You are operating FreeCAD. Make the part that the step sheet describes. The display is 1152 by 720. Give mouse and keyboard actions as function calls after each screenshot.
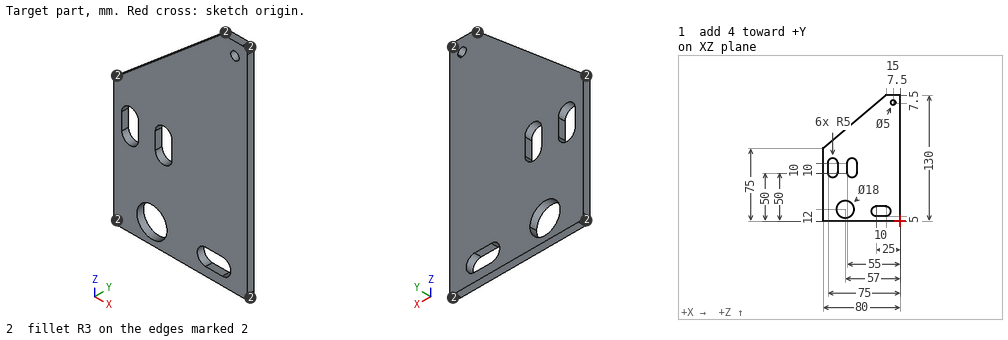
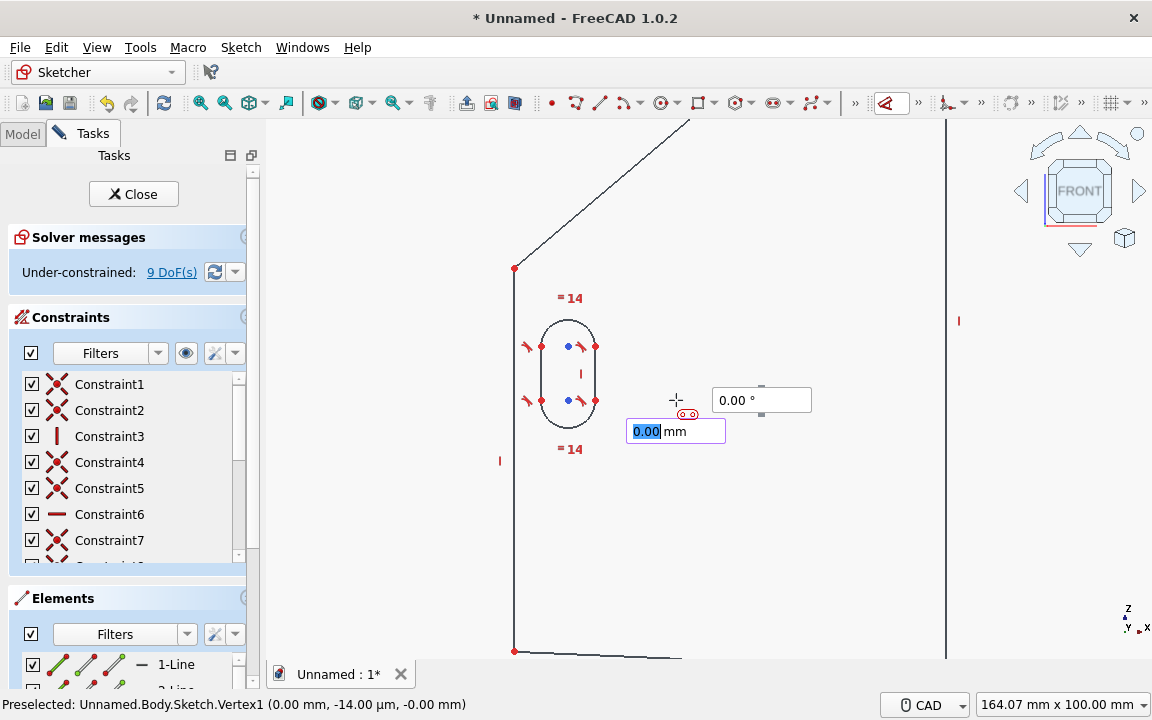
click(676, 346)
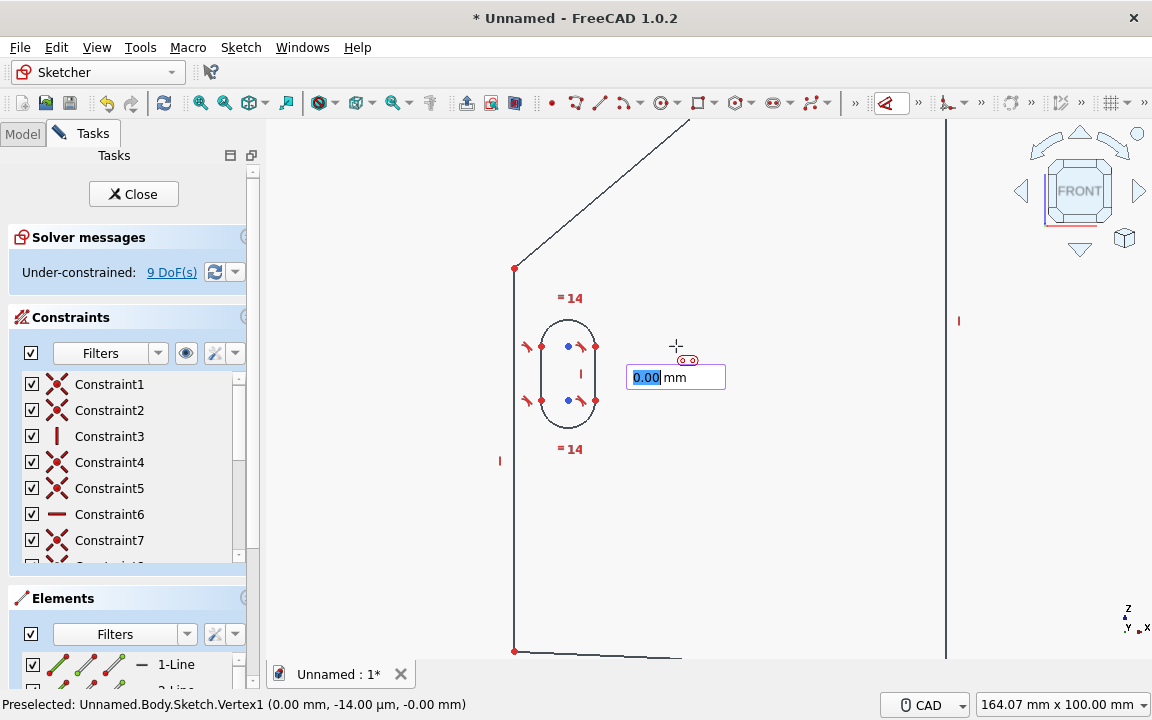
click(703, 373)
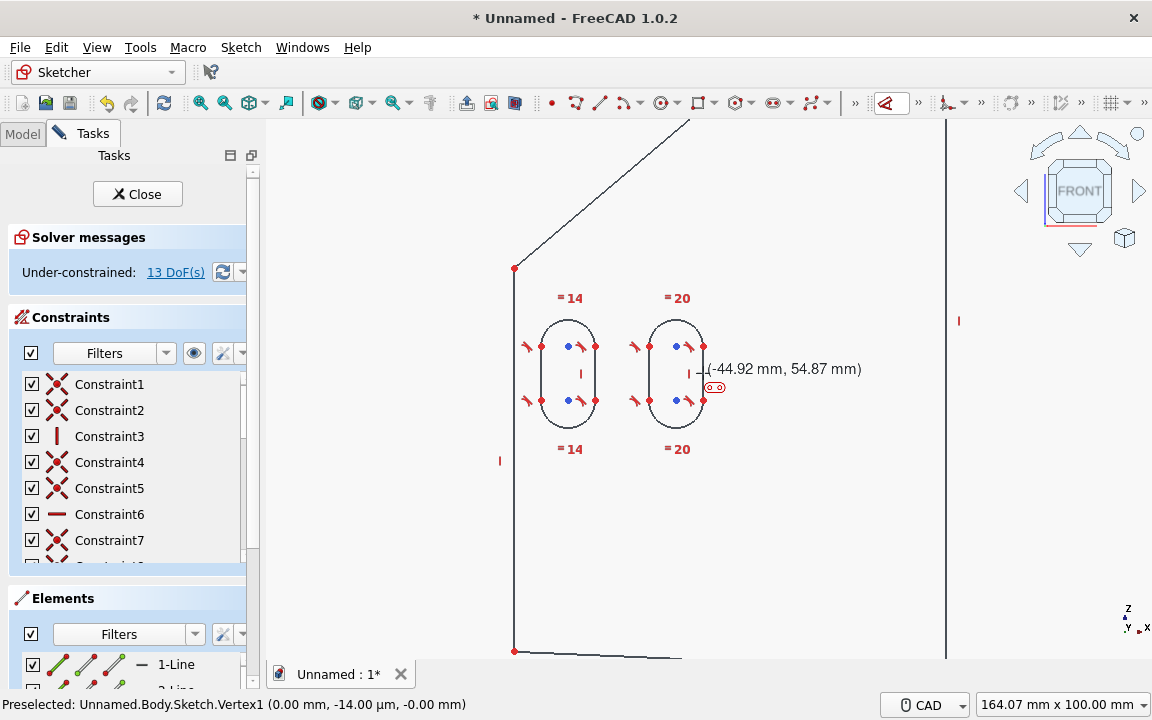
click(811, 616)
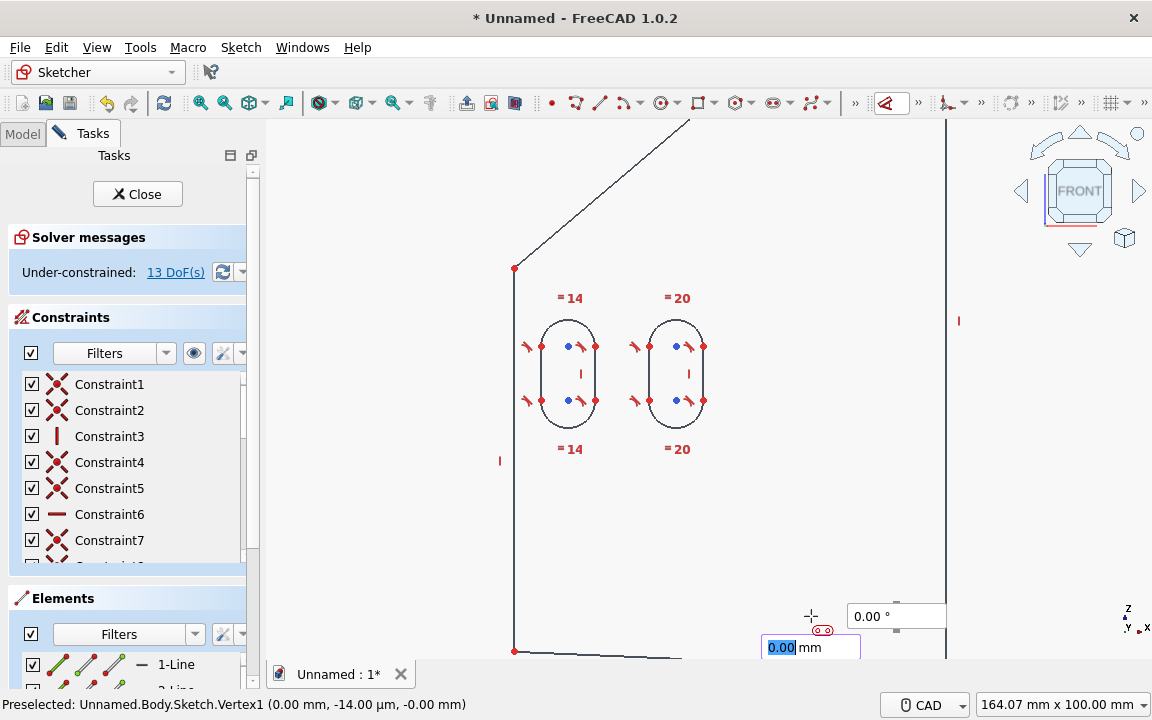
click(865, 616)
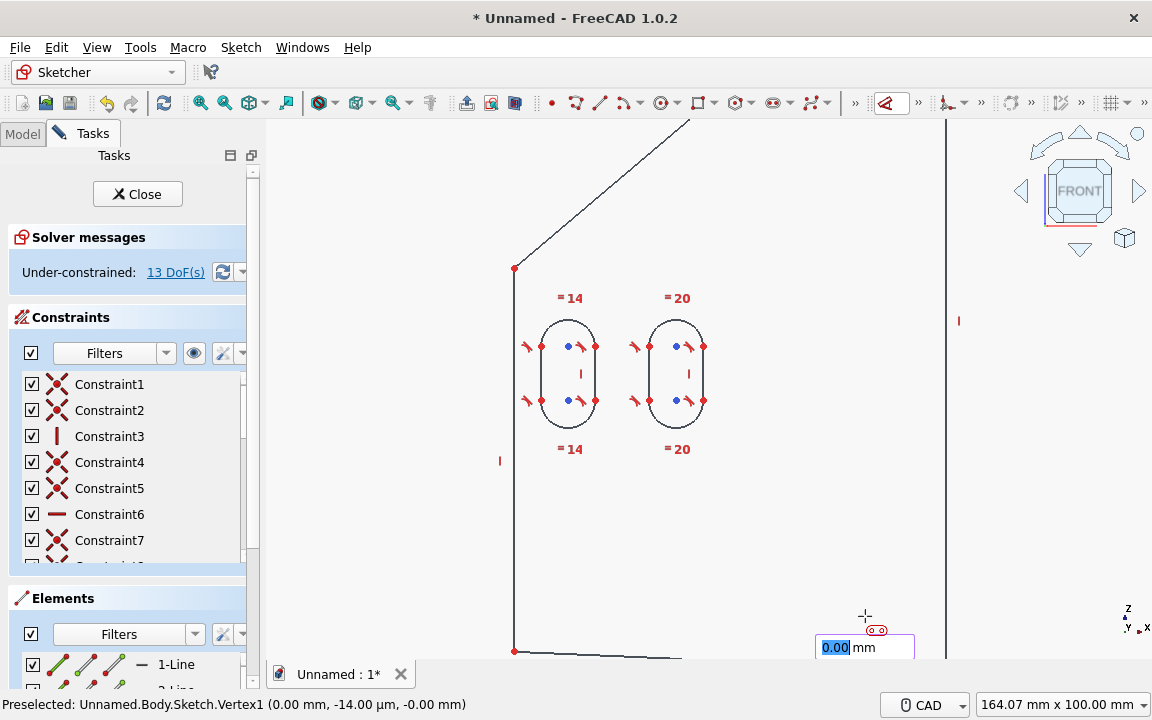
scroll(568, 446, down, 4)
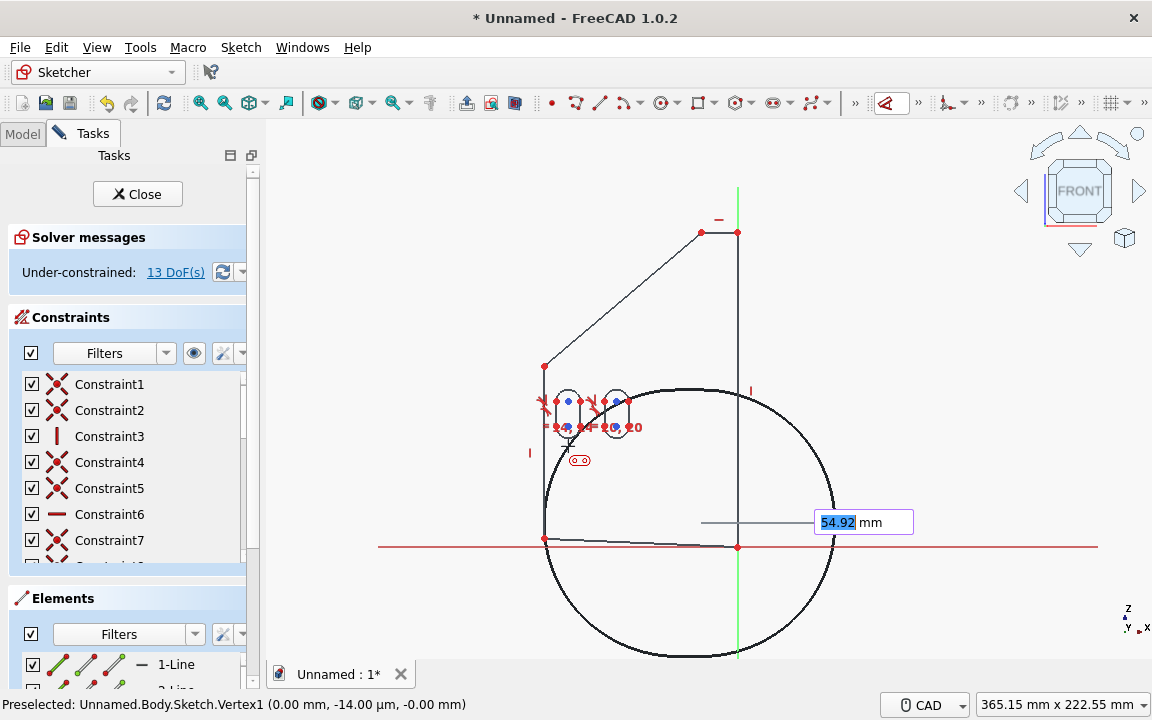
scroll(689, 535, up, 2)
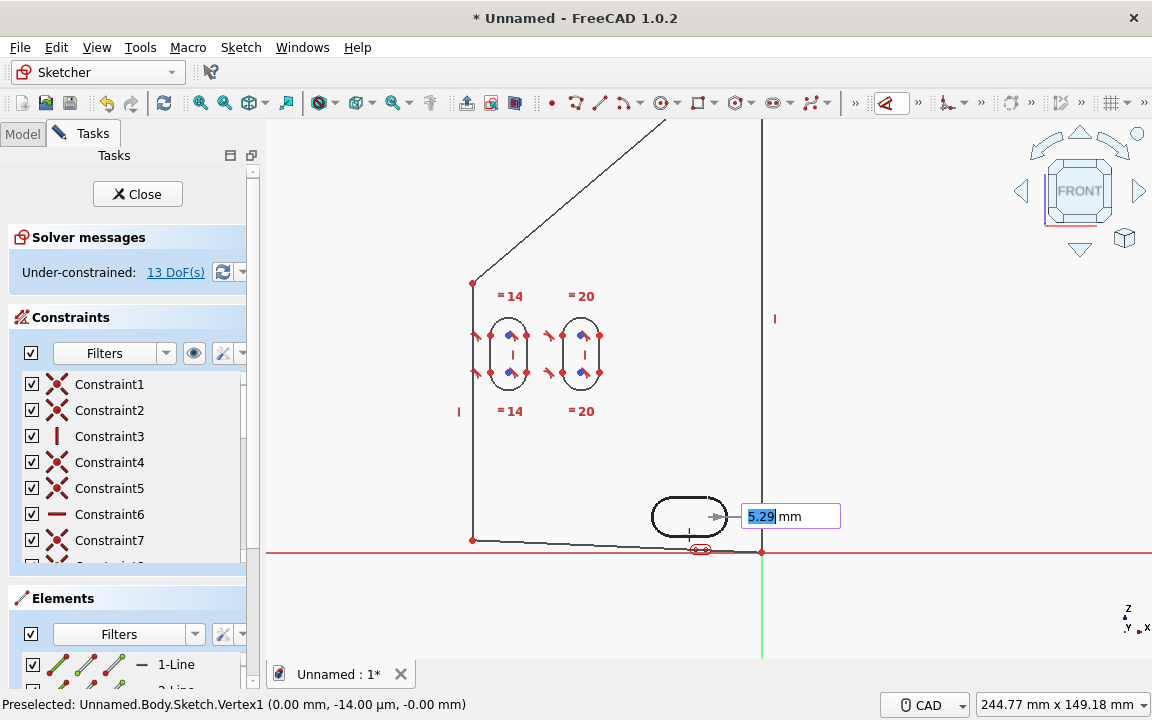
click(689, 535)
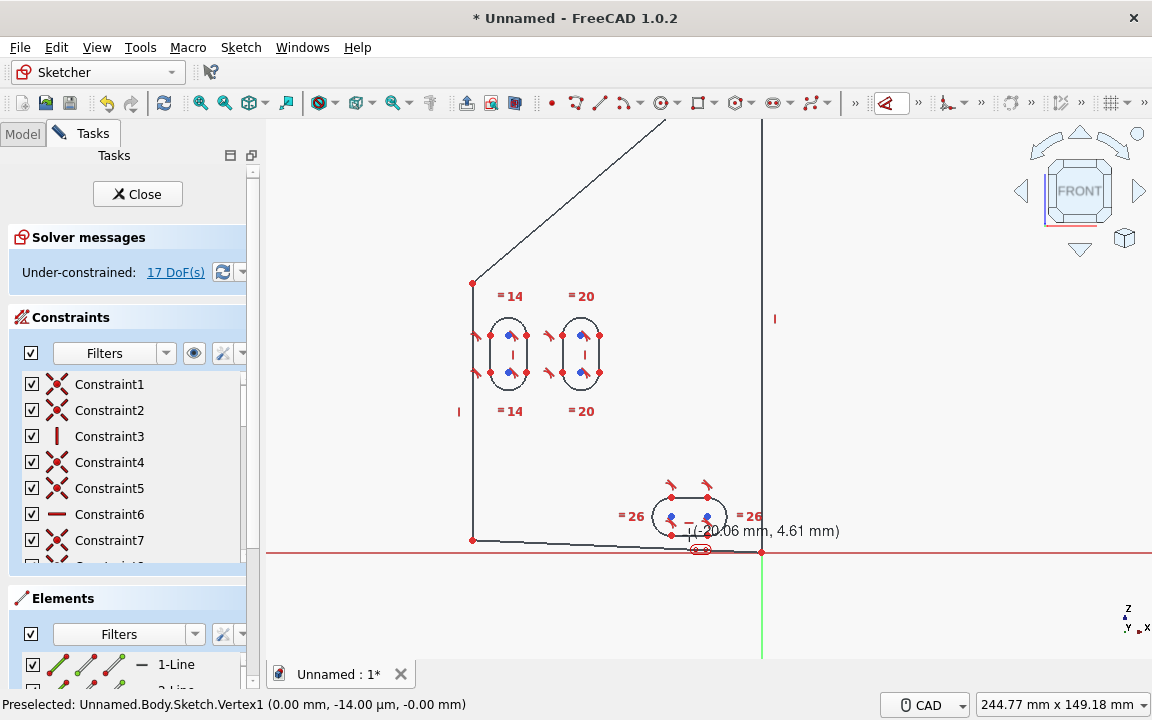
key(g)
key(c)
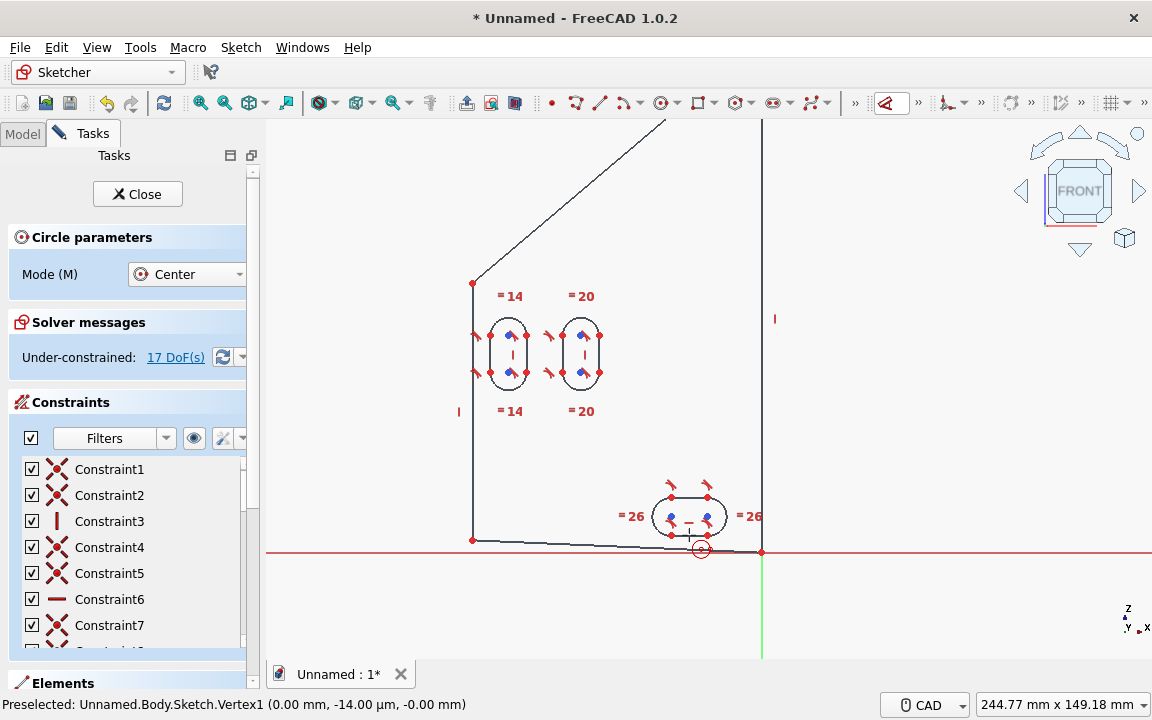
scroll(689, 535, down, 2)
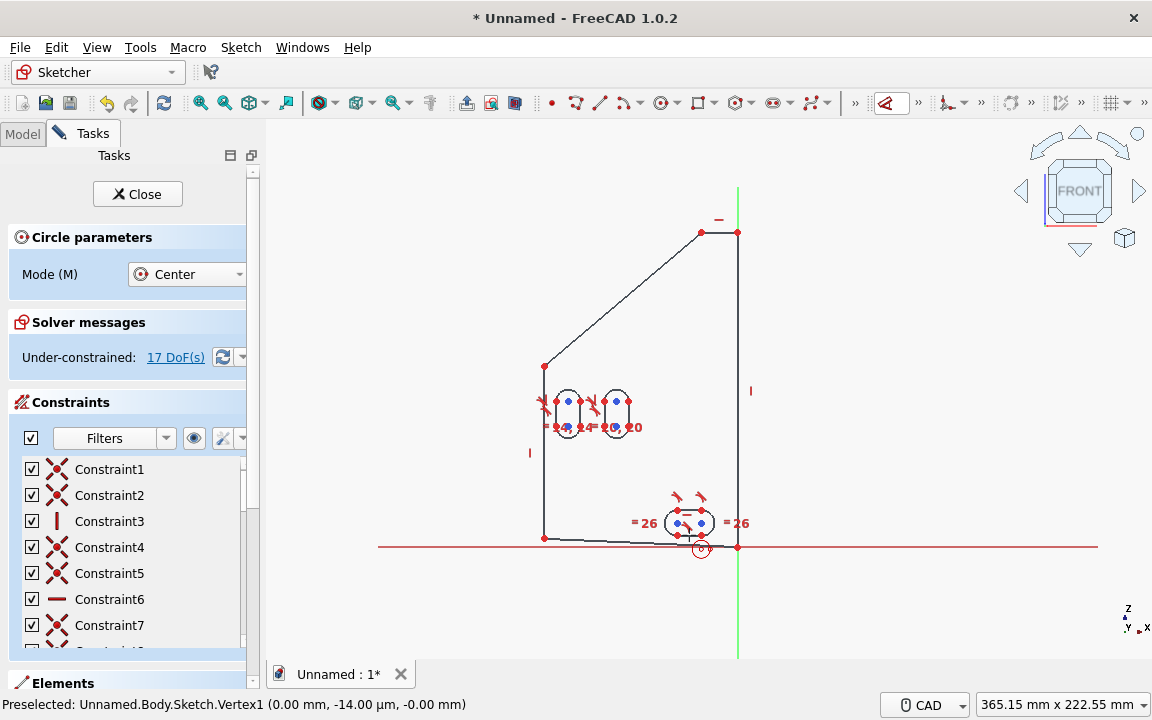
scroll(720, 250, up, 7)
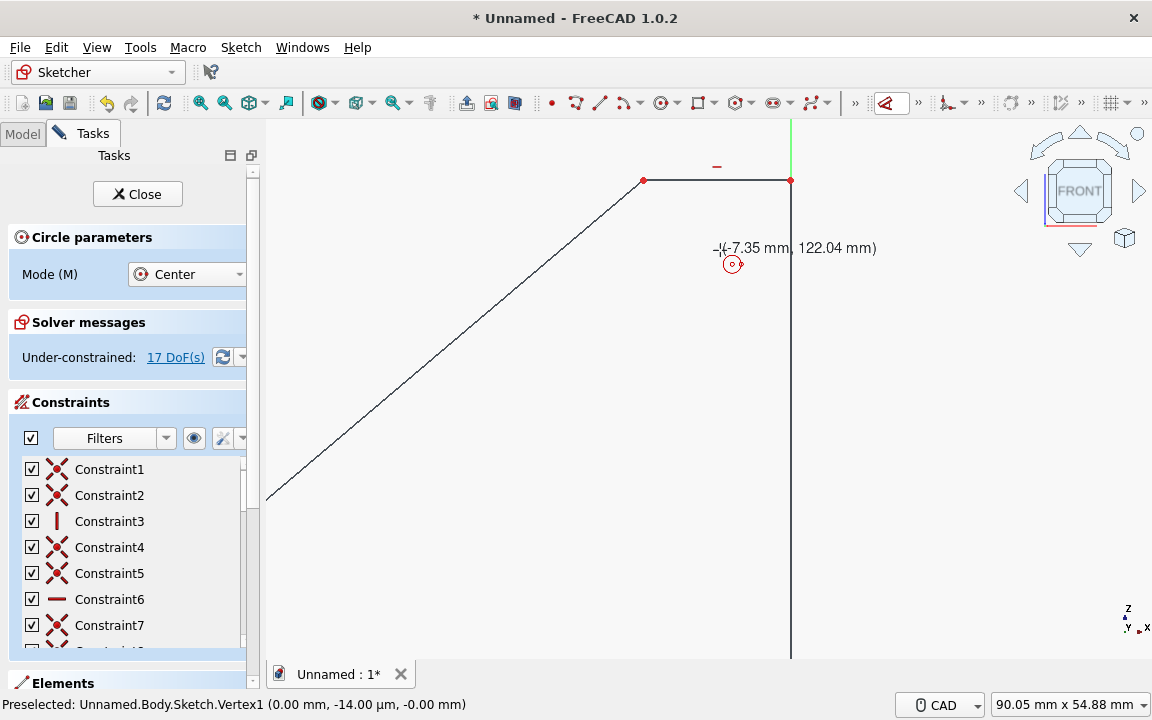
scroll(720, 250, down, 7)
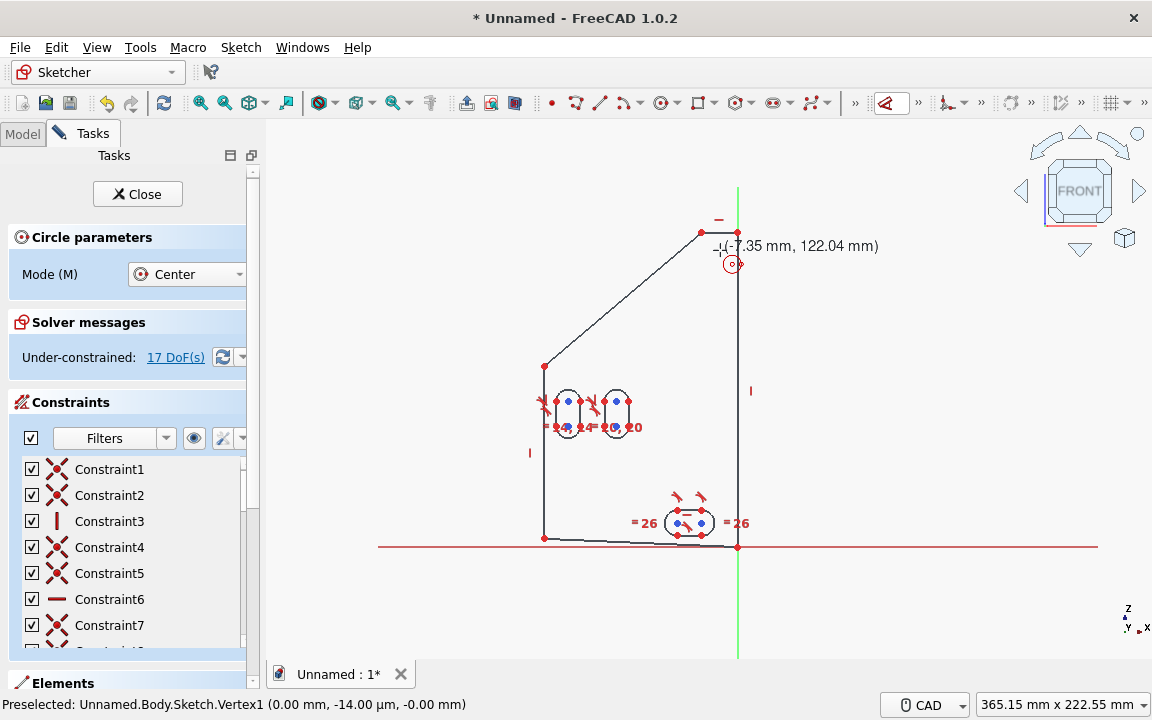
click(720, 250)
move(715, 254)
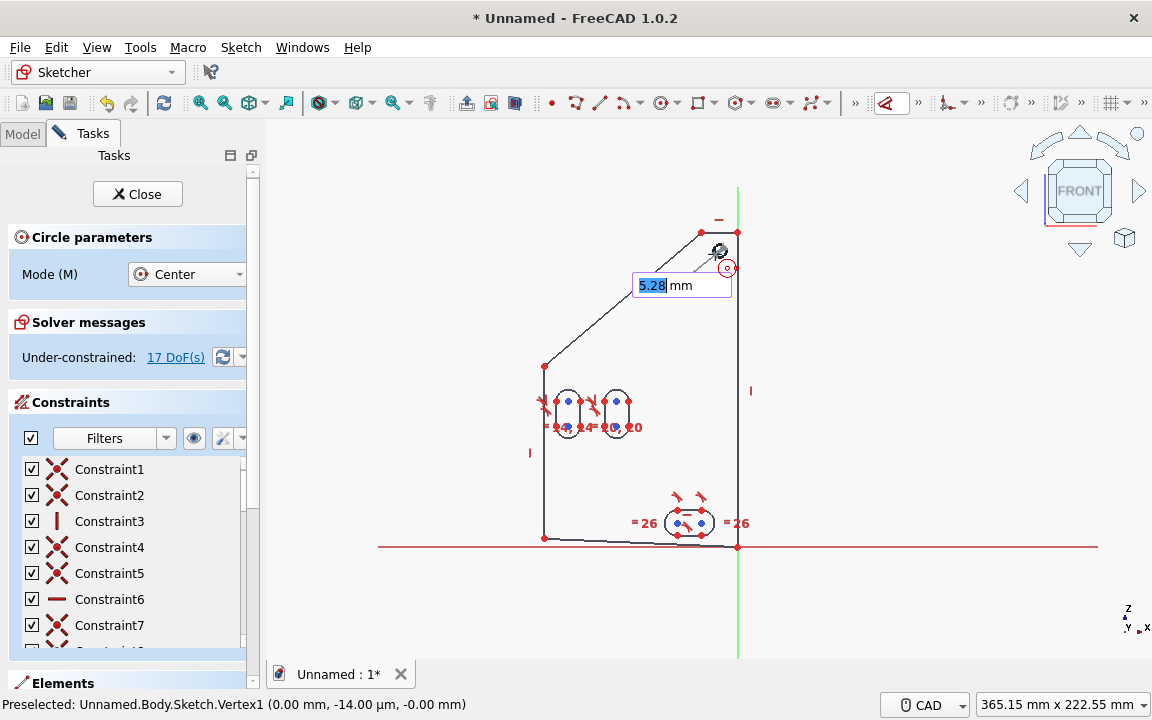
text(5)
key(Return)